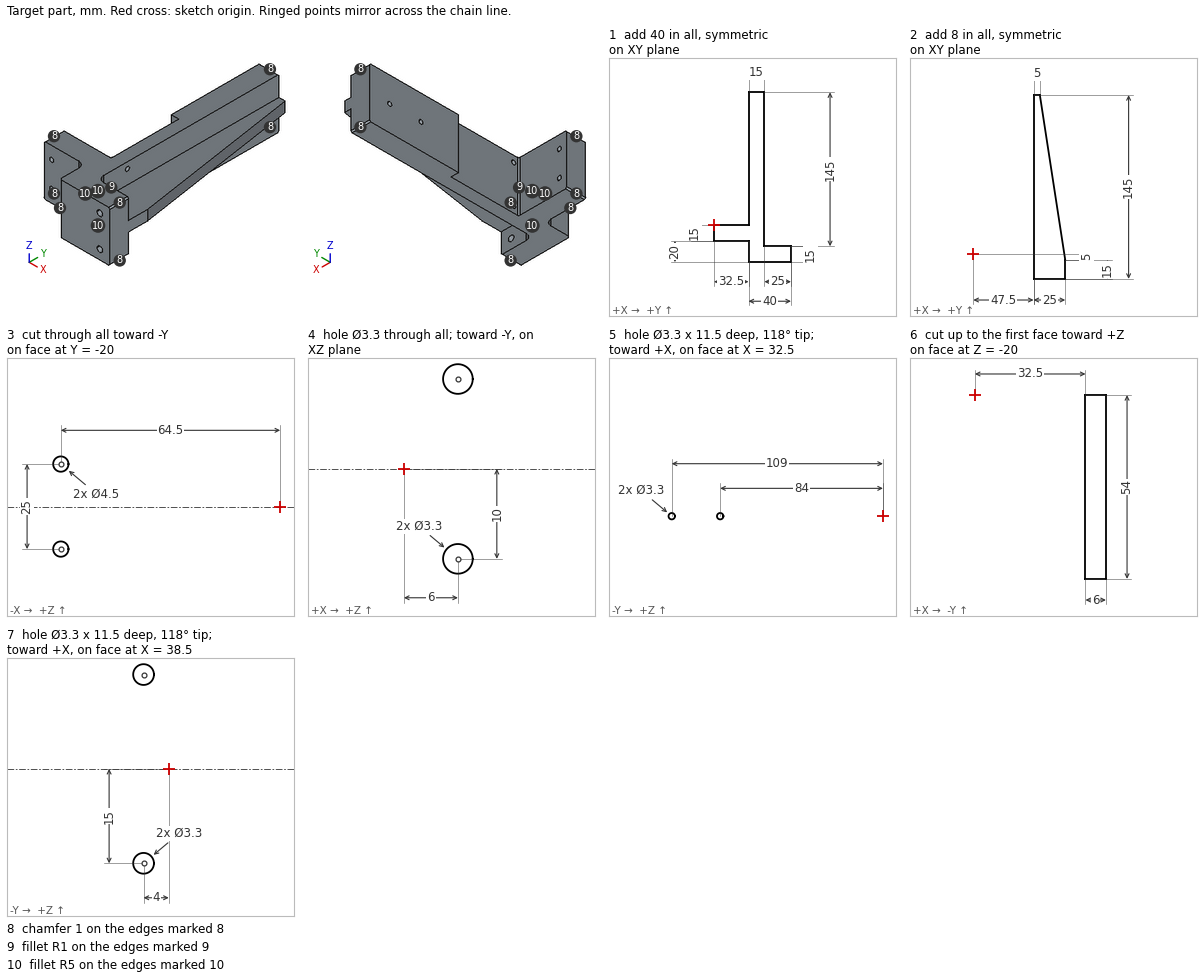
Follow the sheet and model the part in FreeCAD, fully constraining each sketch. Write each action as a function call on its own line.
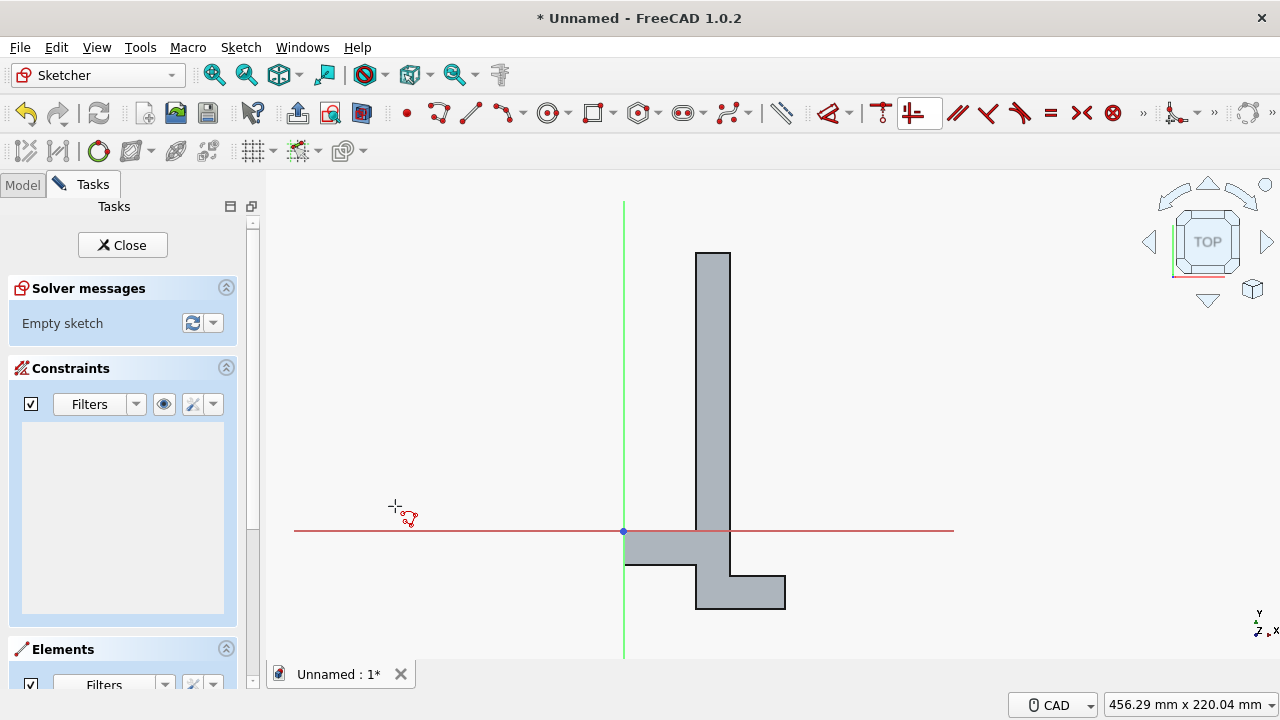
click(730, 576)
click(785, 576)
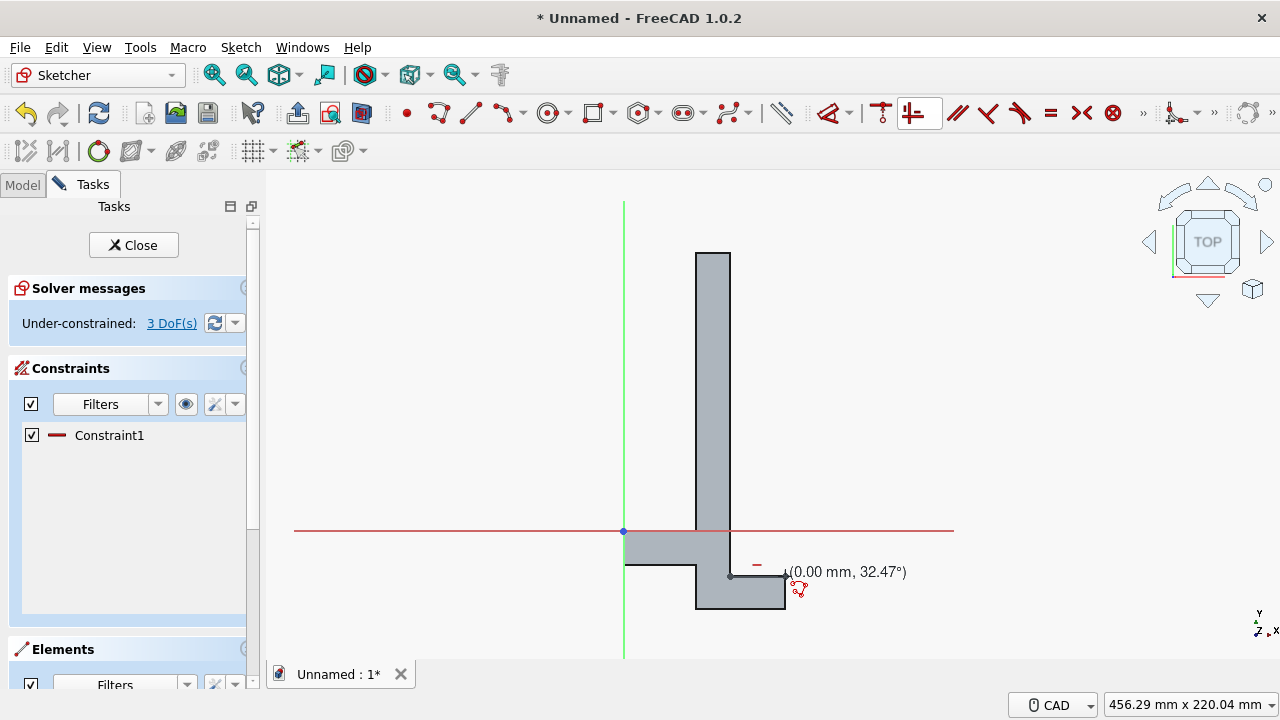
scroll(785, 542, up, 2)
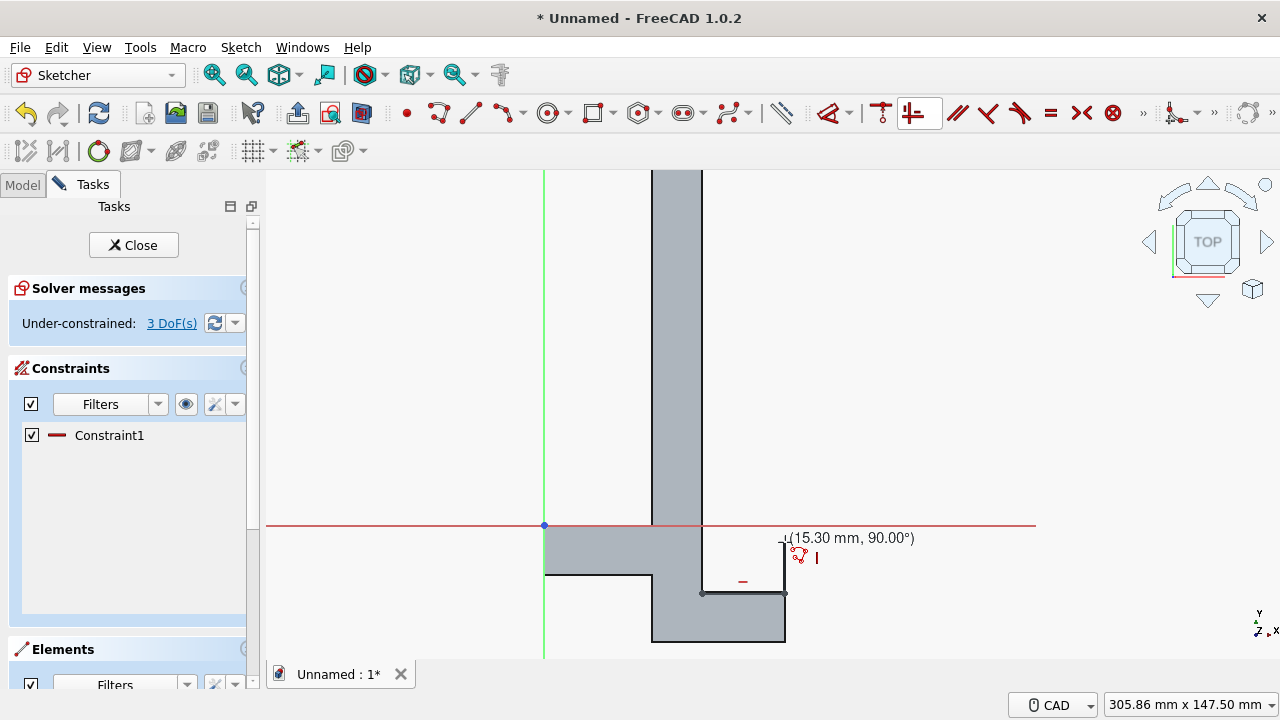
click(785, 542)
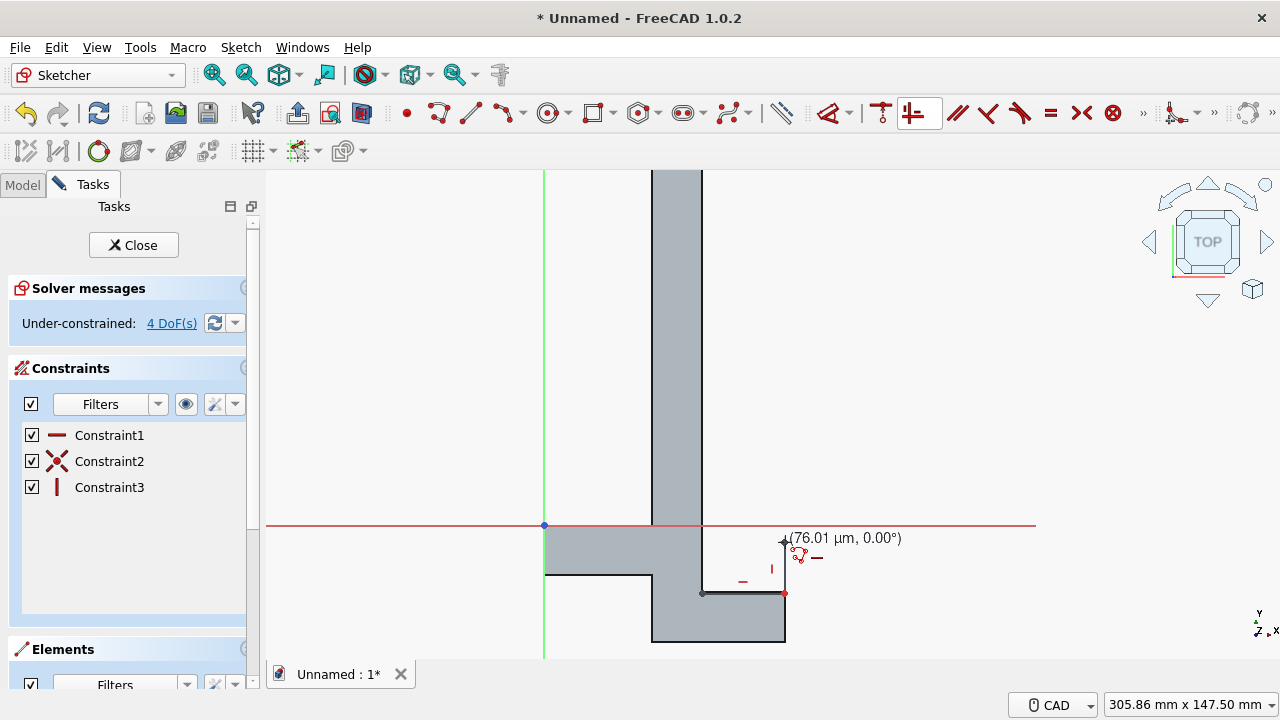
scroll(786, 543, down, 2)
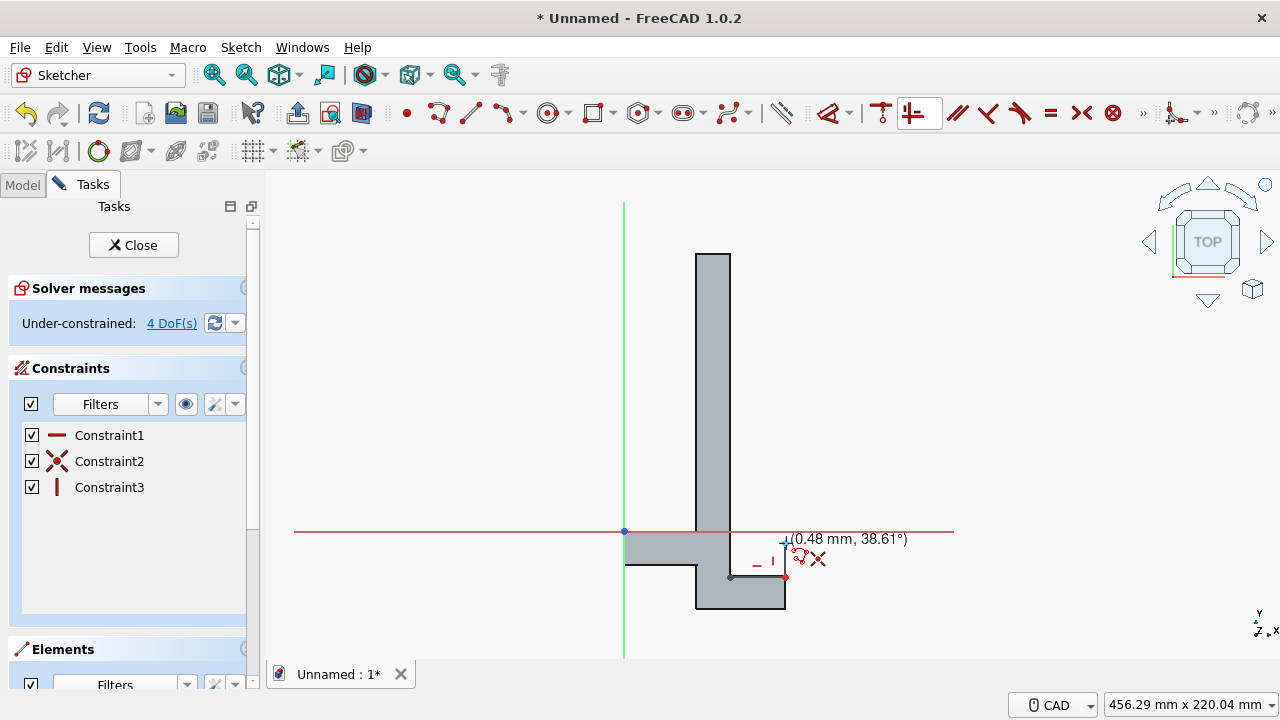
click(741, 254)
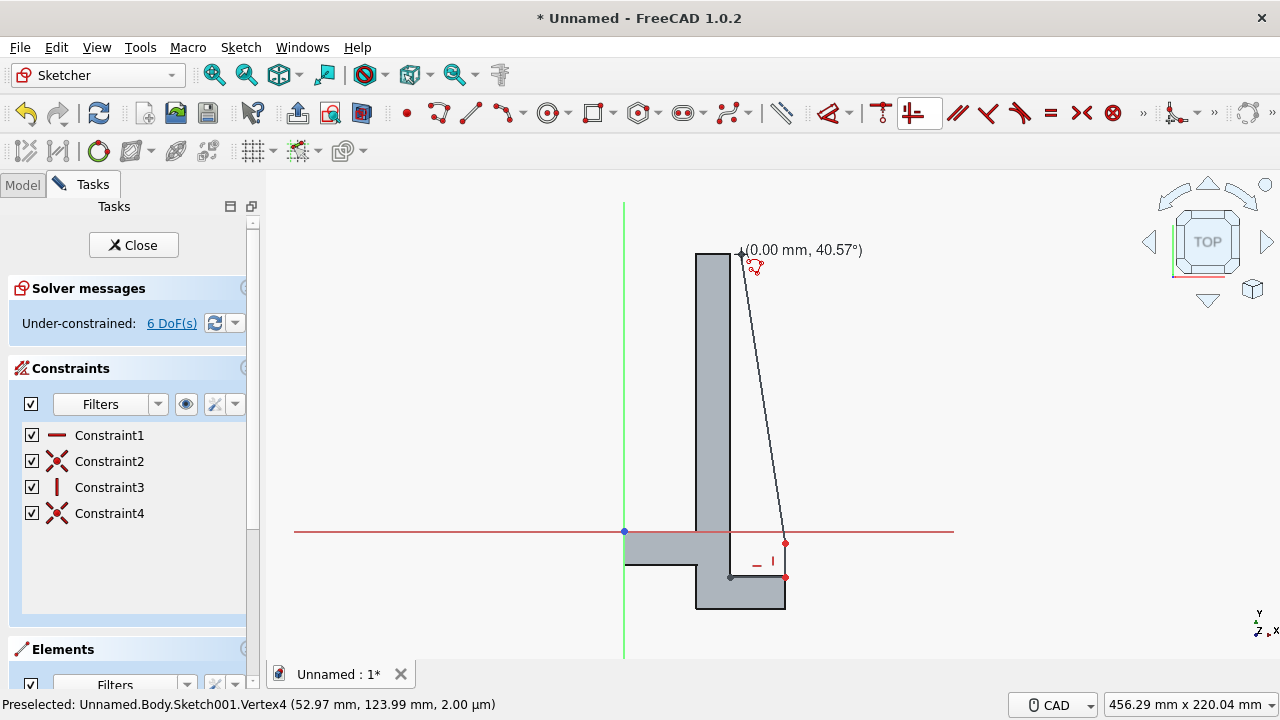
scroll(730, 254, up, 2)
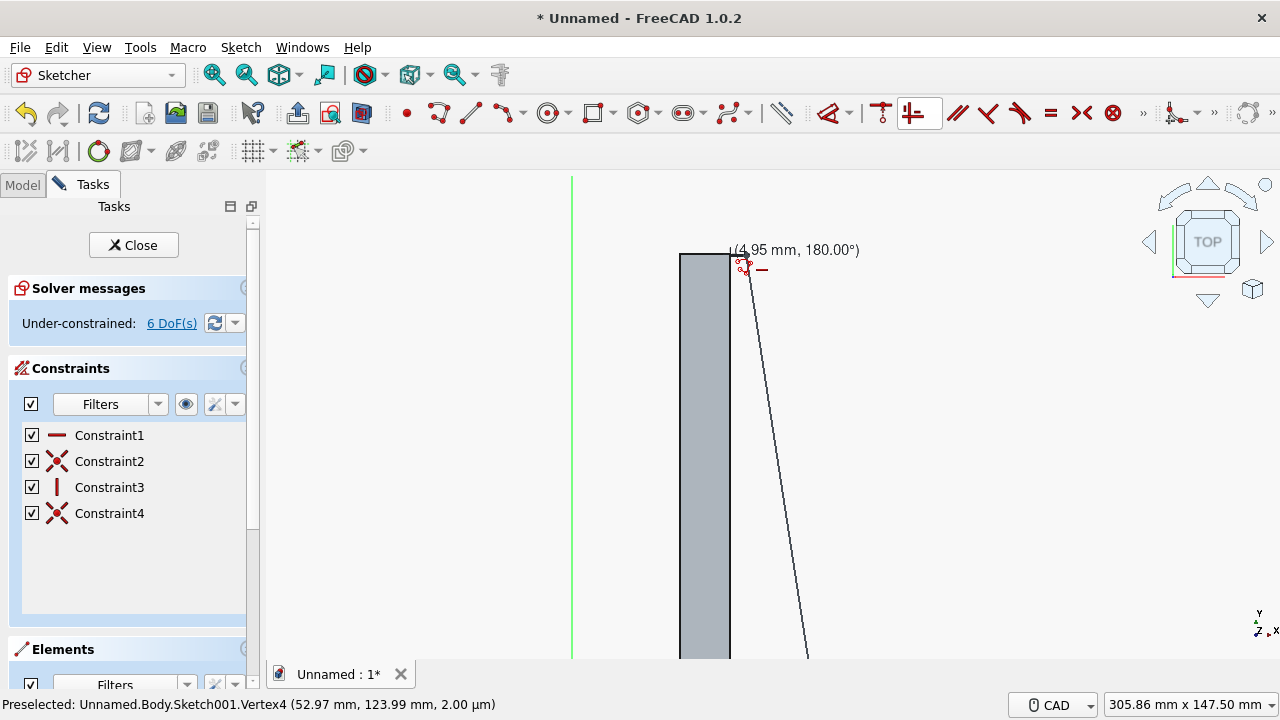
click(730, 254)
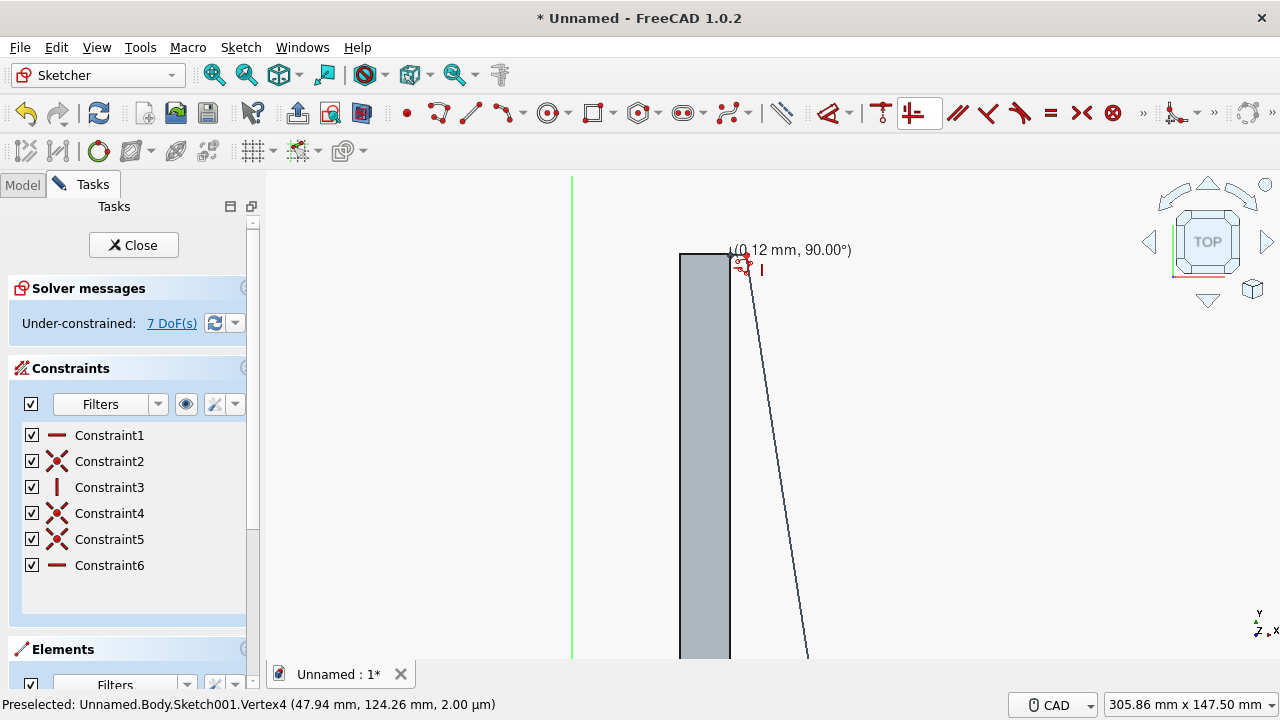
scroll(729, 253, down, 2)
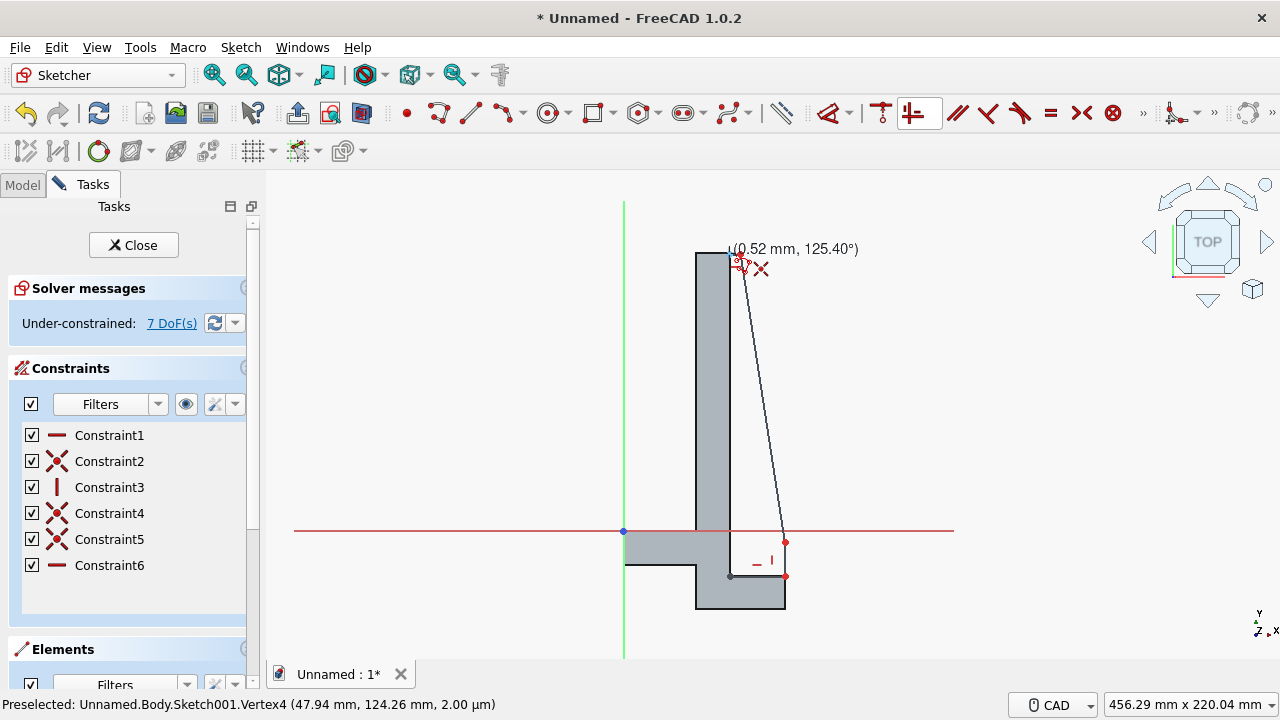
click(730, 577)
key(Escape)
key(Escape)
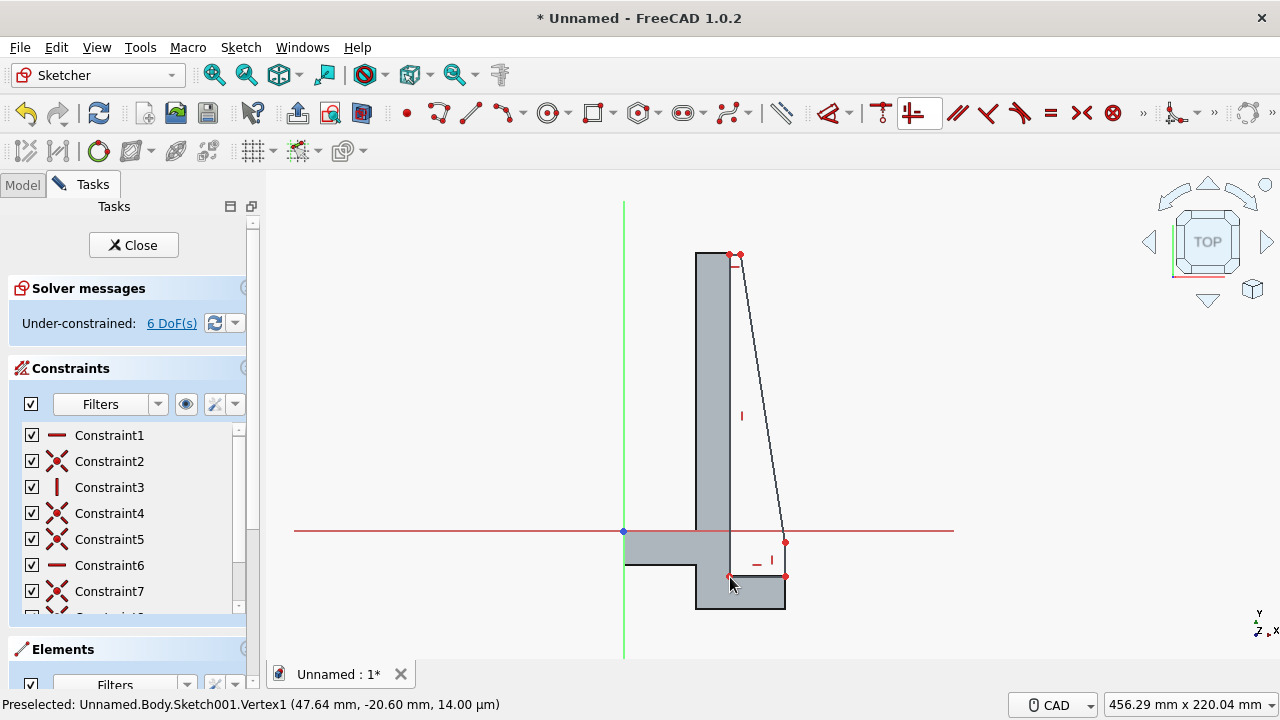
click(828, 114)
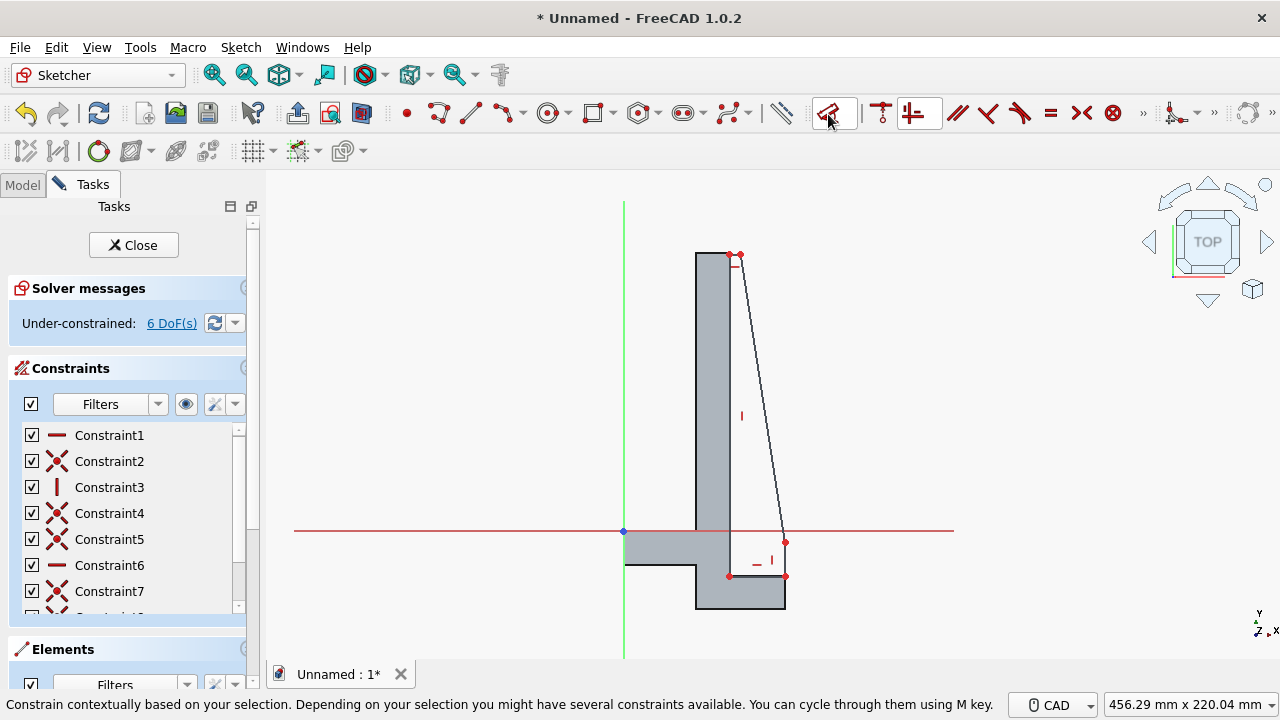
scroll(735, 255, up, 7)